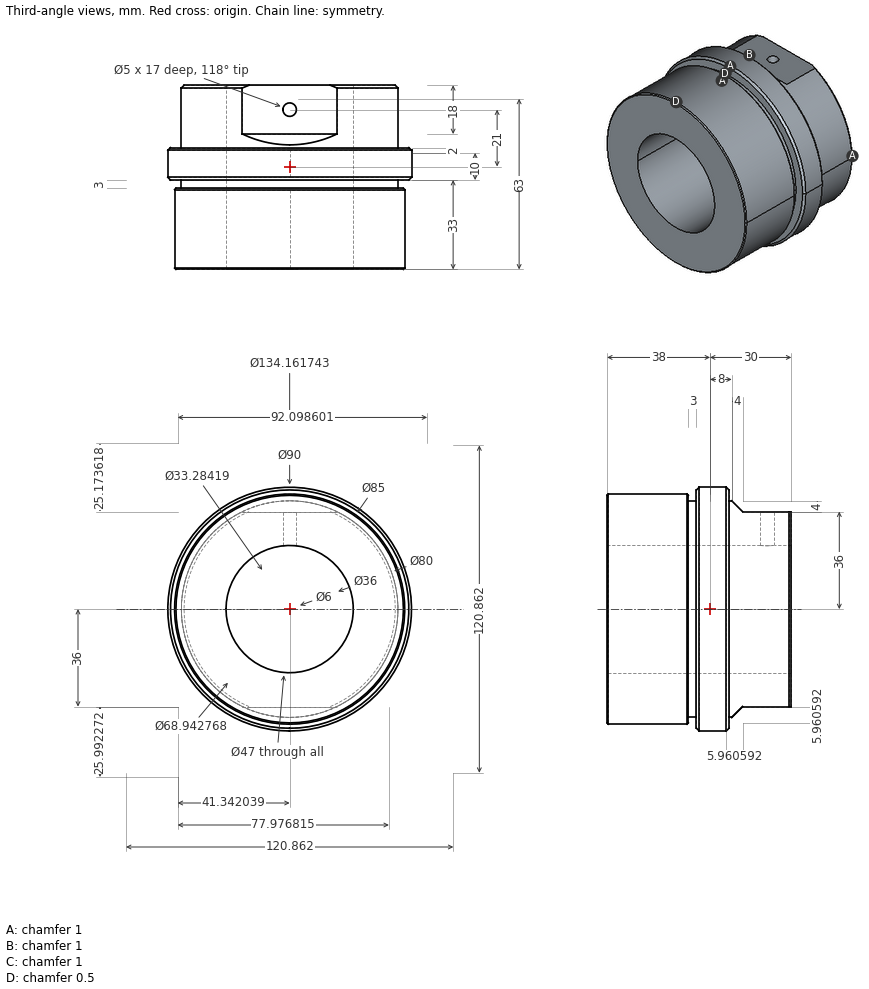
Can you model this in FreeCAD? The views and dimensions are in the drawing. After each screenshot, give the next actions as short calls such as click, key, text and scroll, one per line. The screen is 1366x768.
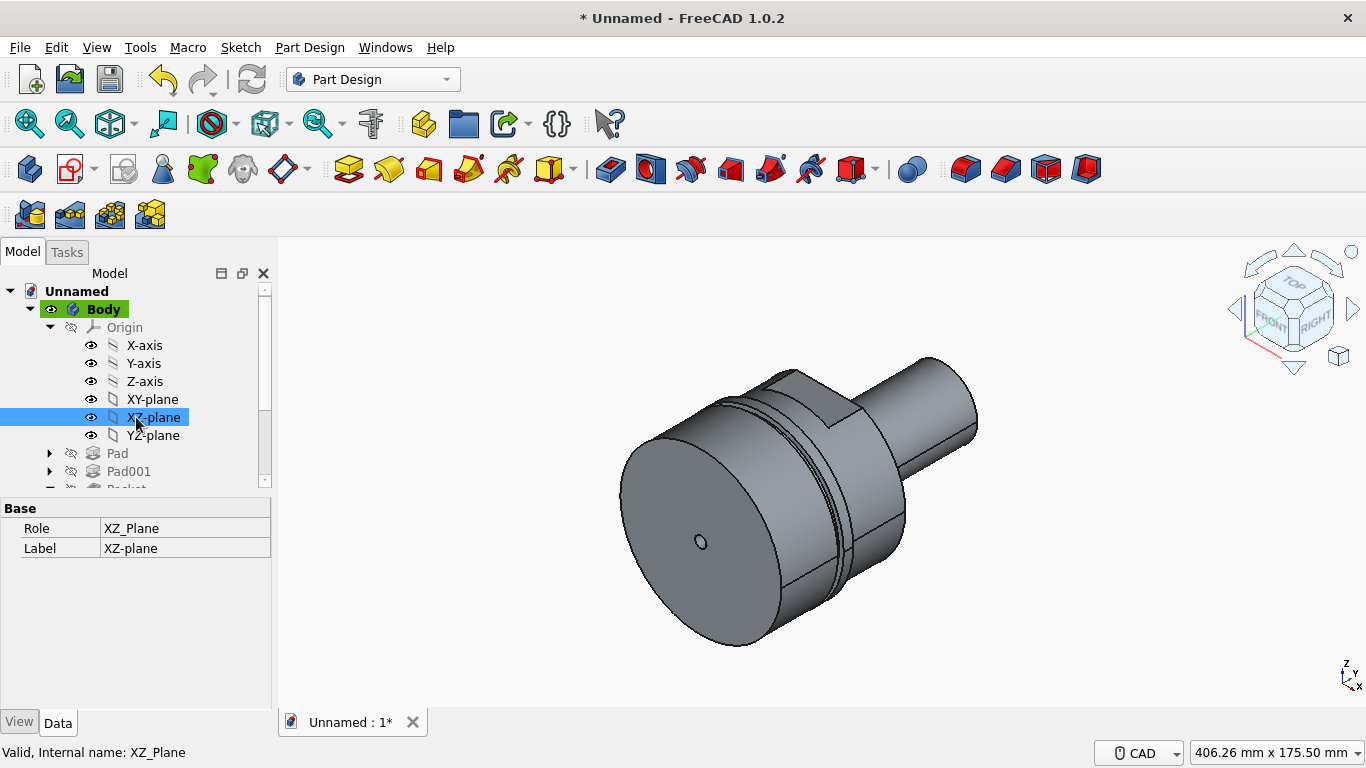
click(284, 170)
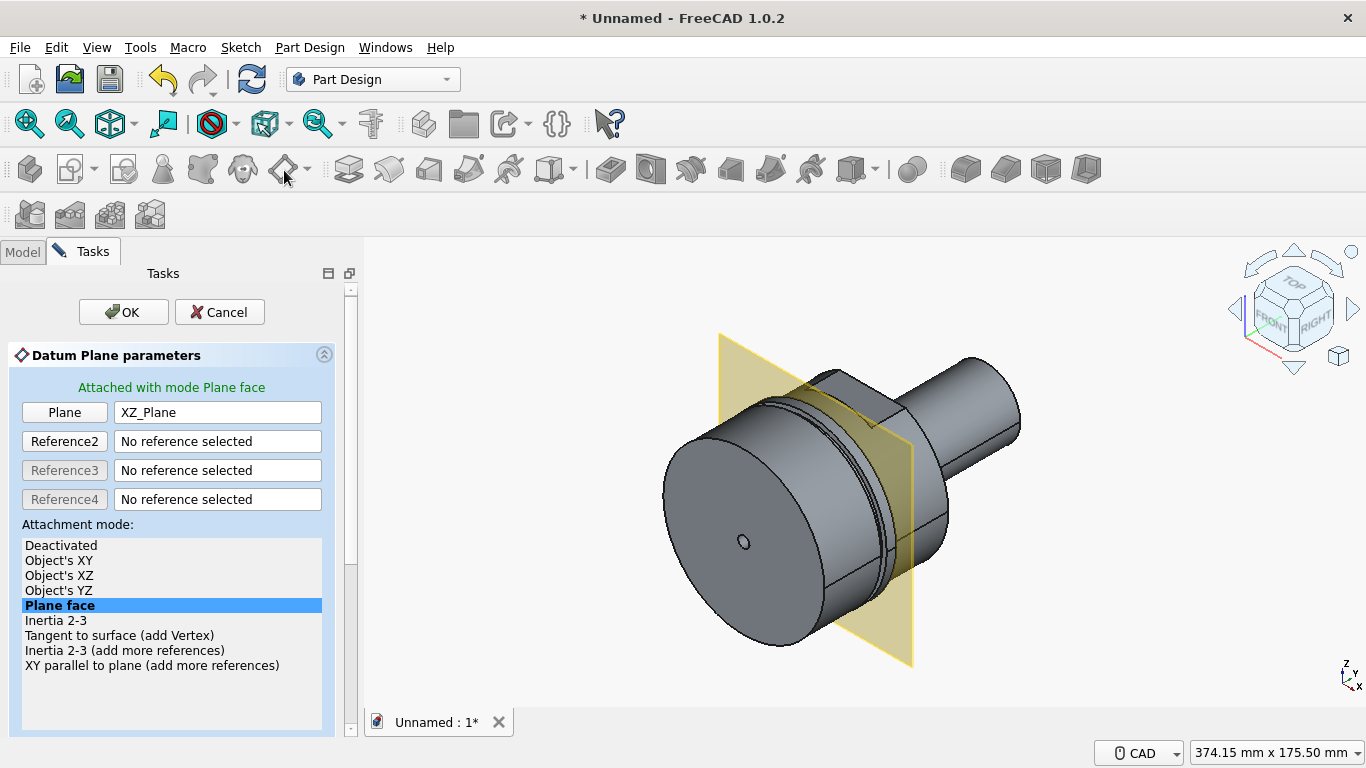
scroll(351, 510, down, 3)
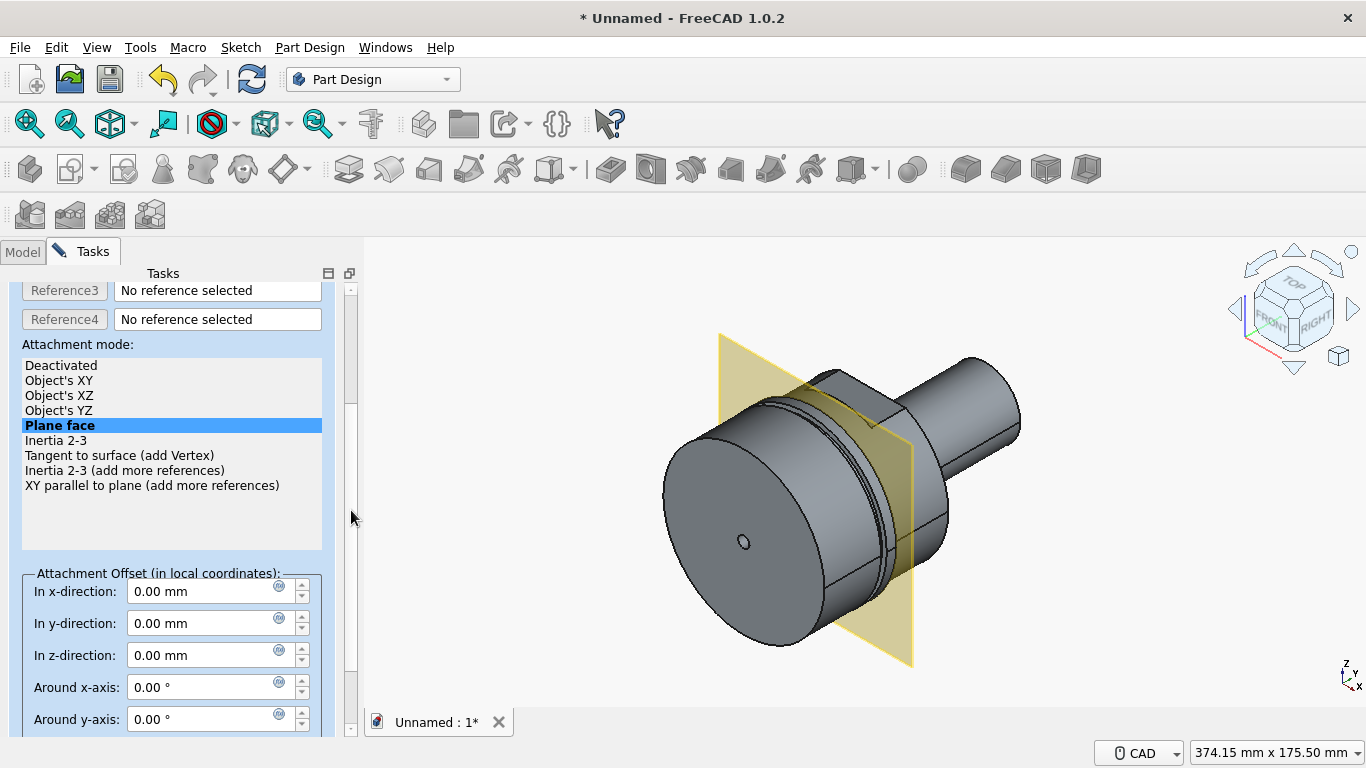
triple_click(210, 655)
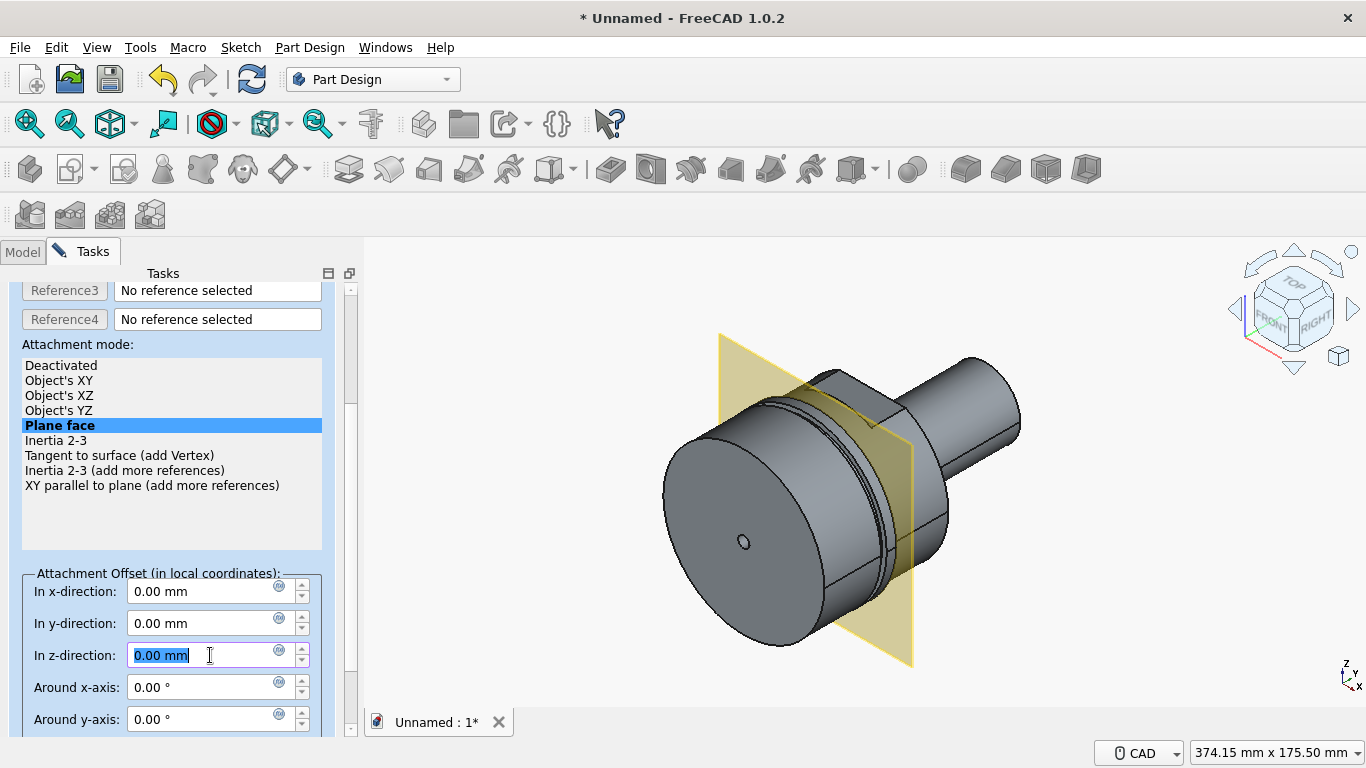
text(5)
key(Tab)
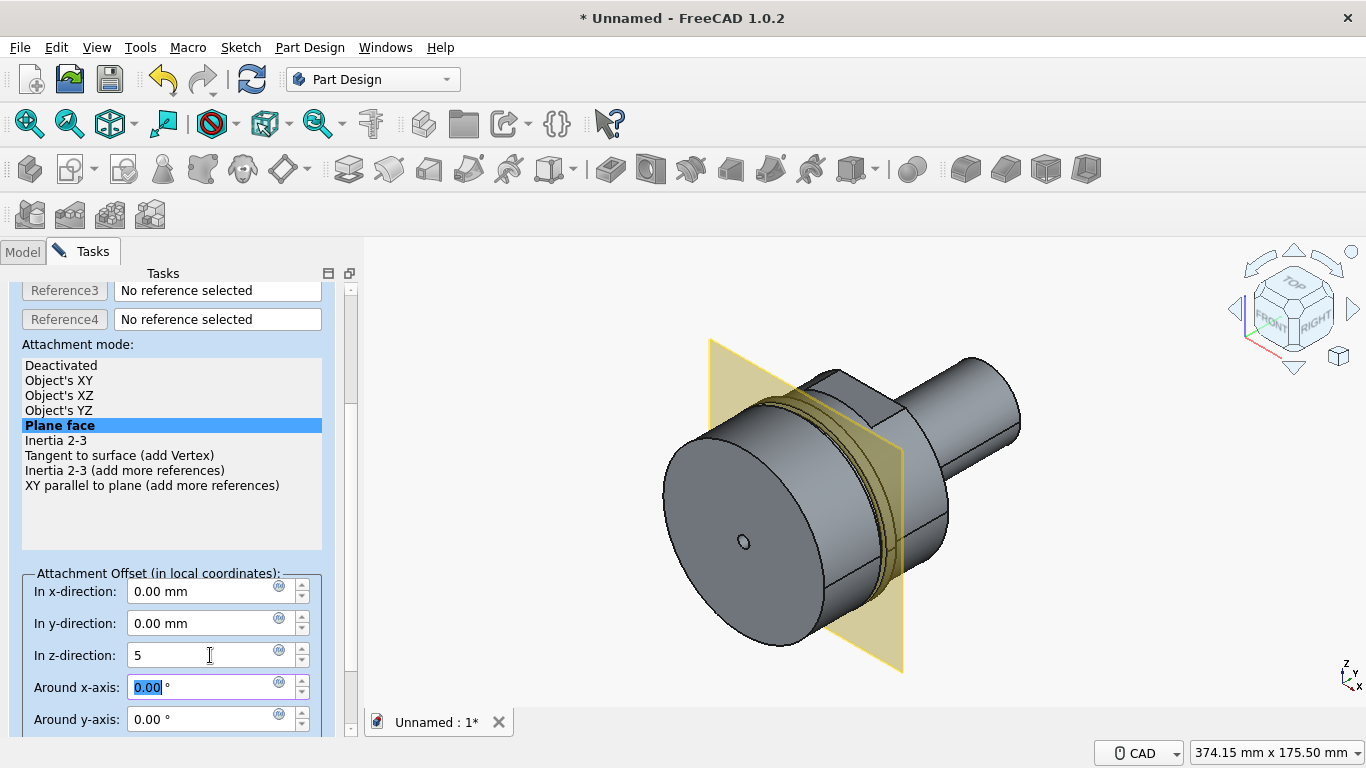
scroll(351, 510, up, 4)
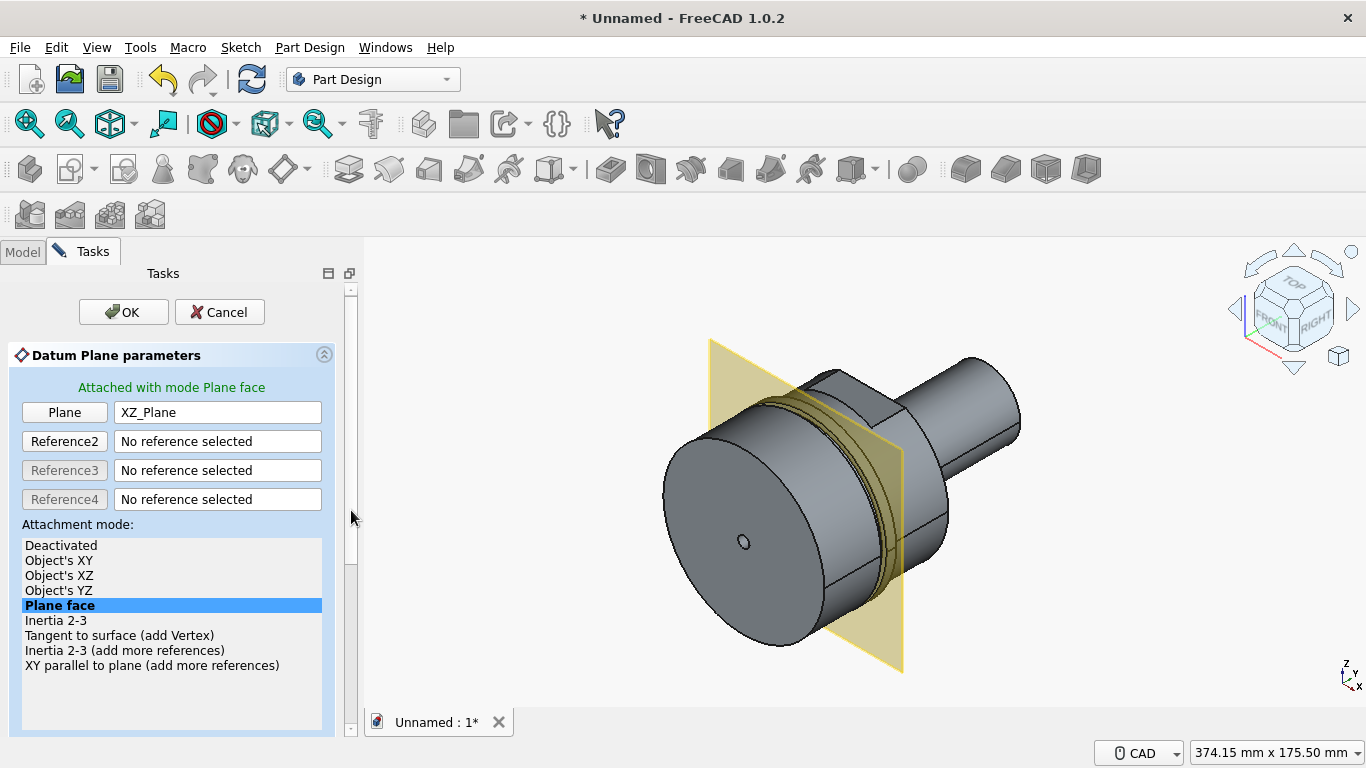
click(124, 312)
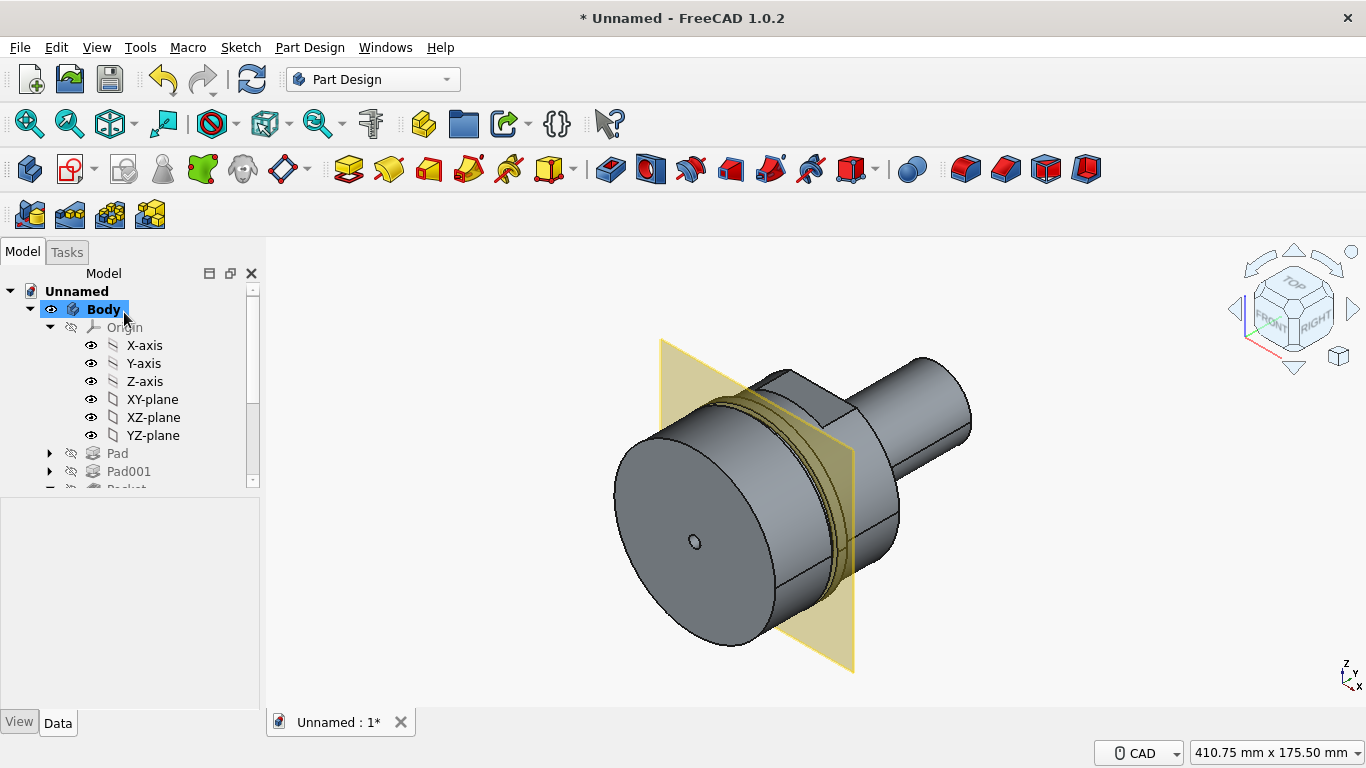
scroll(100, 377, down, 3)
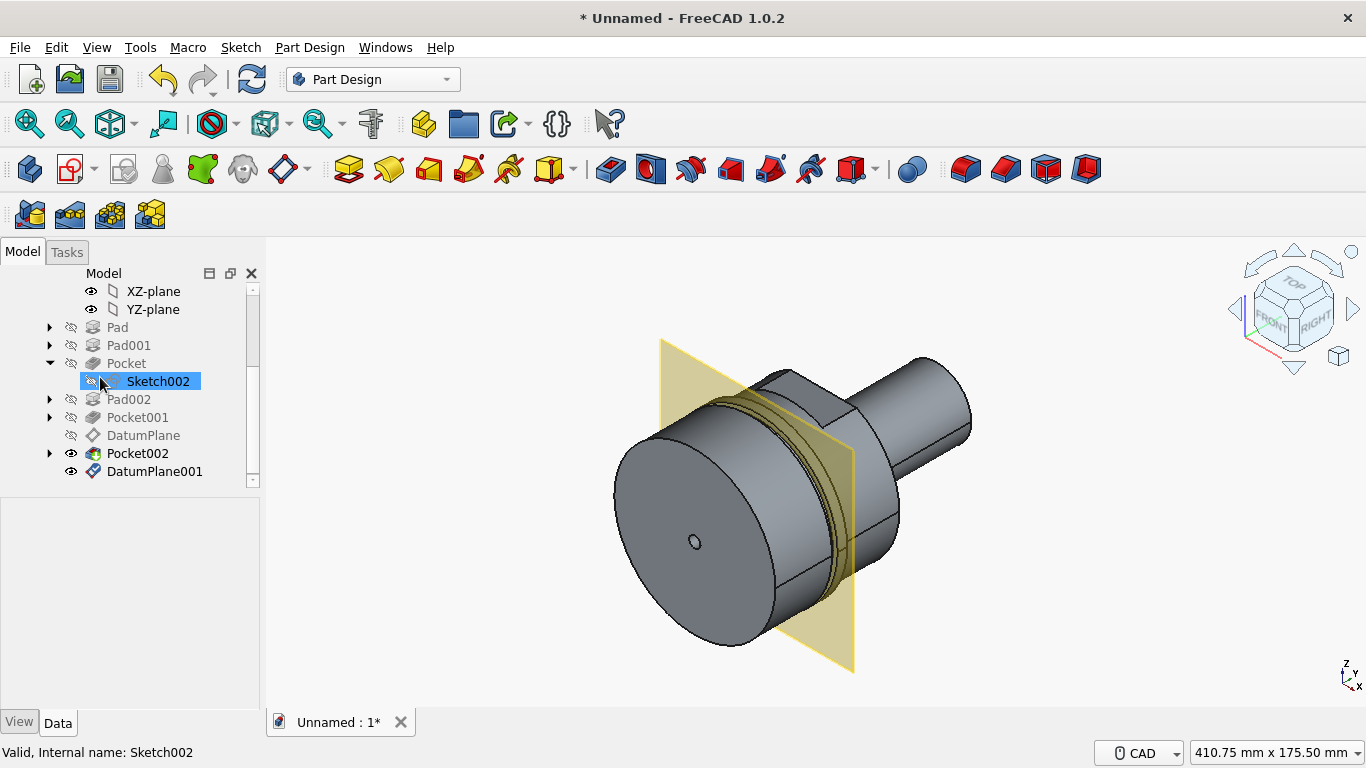
click(116, 471)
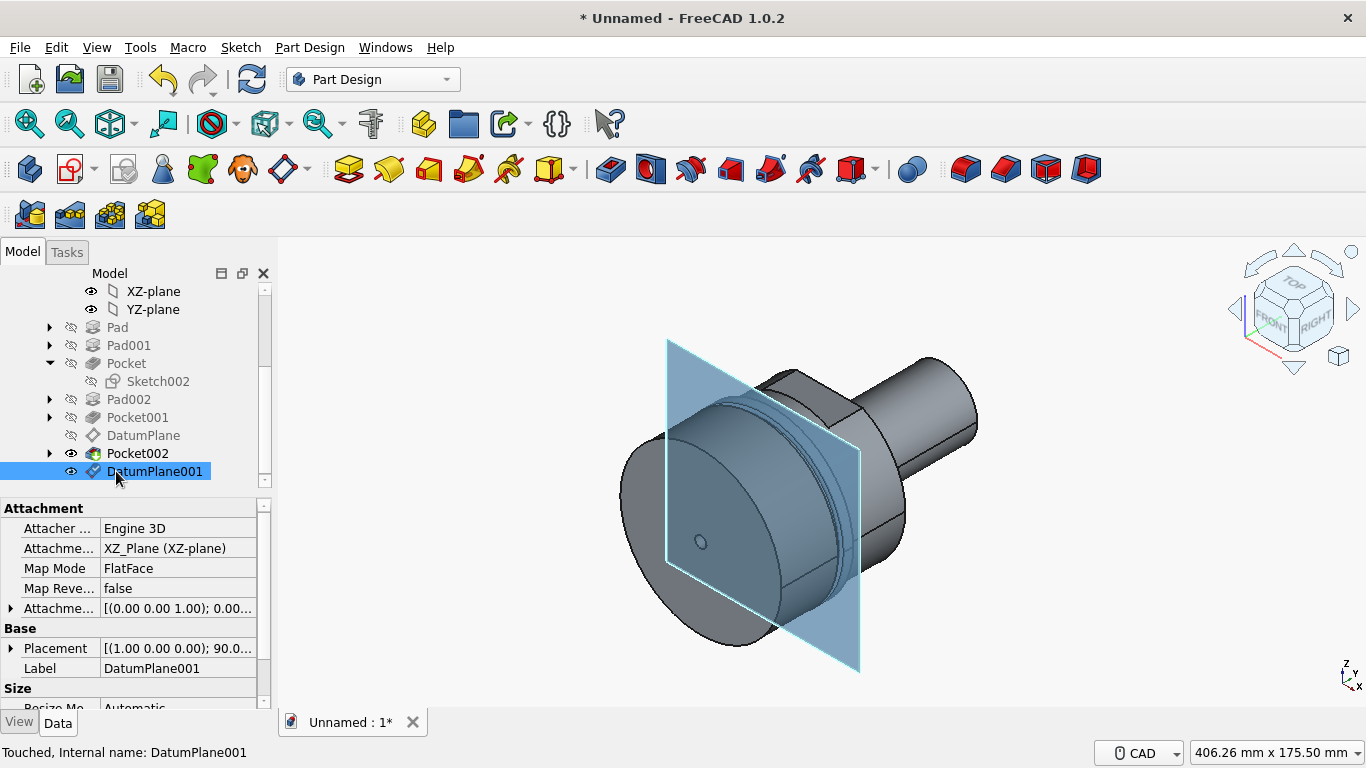
click(70, 170)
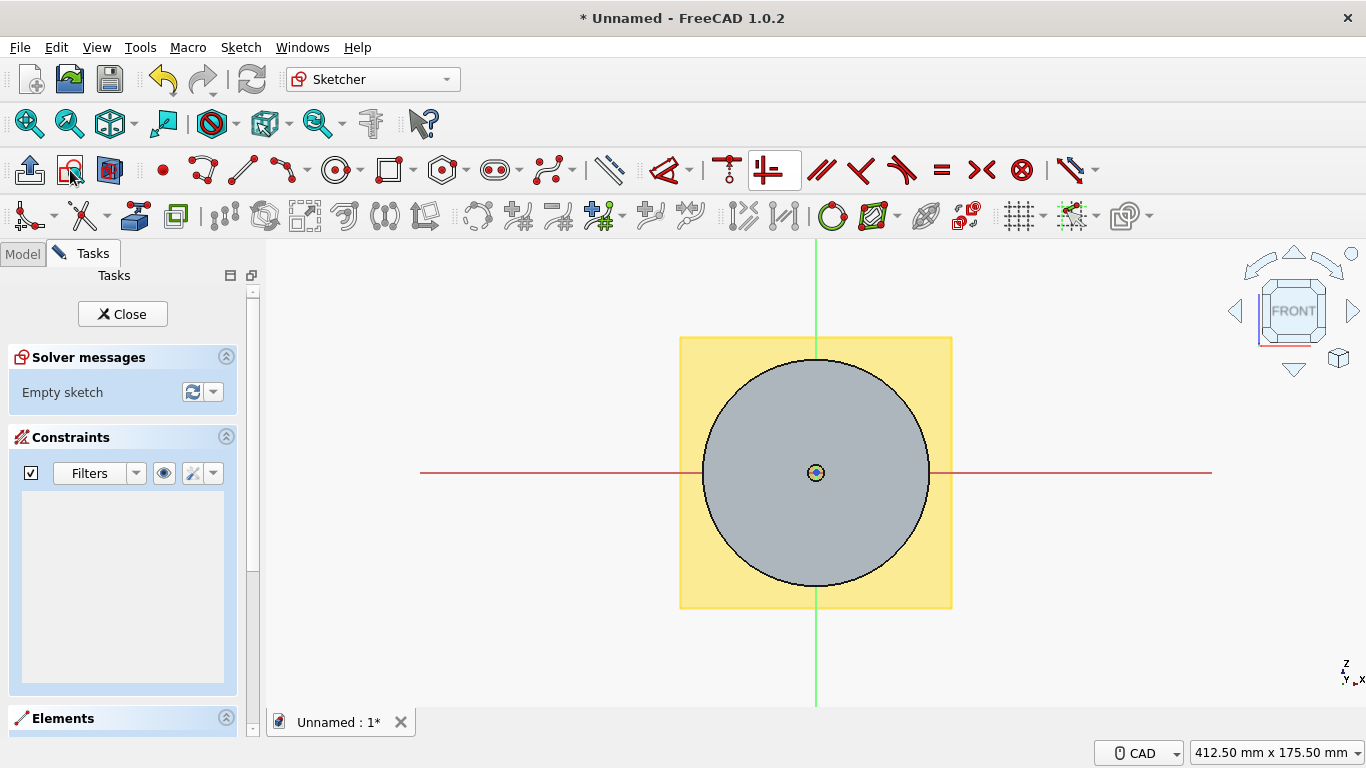
click(110, 170)